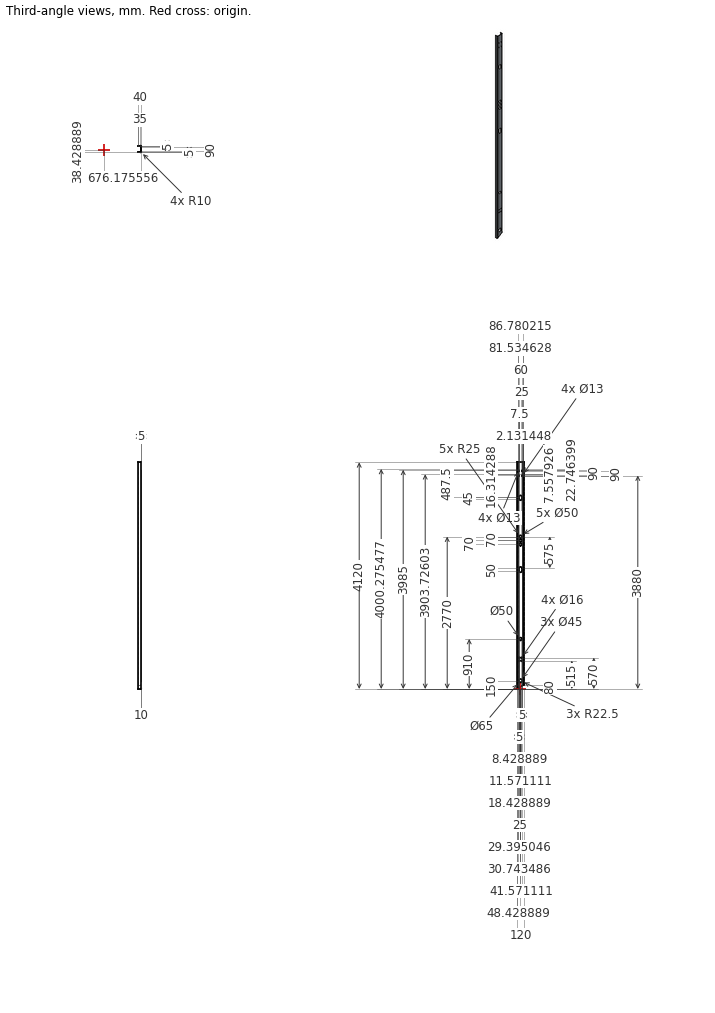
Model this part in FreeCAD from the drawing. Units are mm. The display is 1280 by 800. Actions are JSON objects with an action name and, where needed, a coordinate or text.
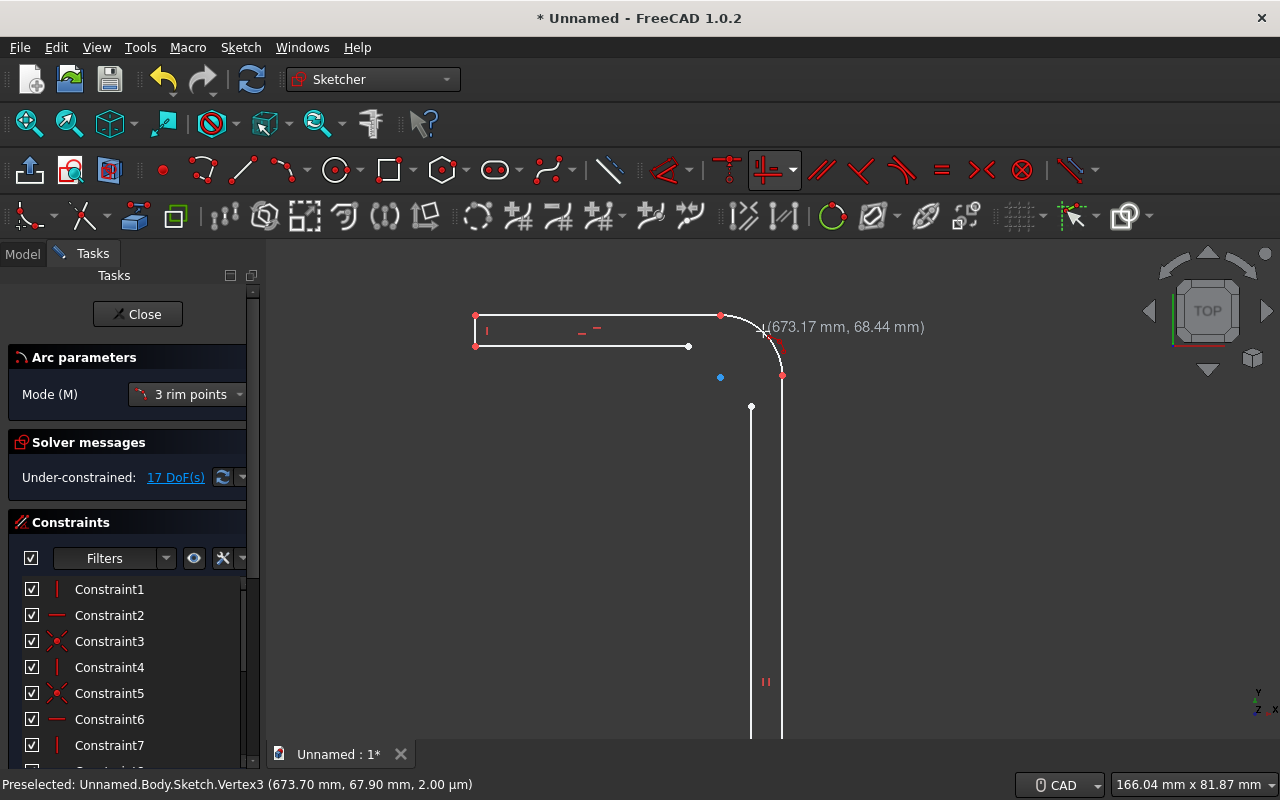
{"action": "left_click", "coordinate": [689, 346]}
{"action": "left_click", "coordinate": [751, 406]}
{"action": "left_click", "coordinate": [733, 361]}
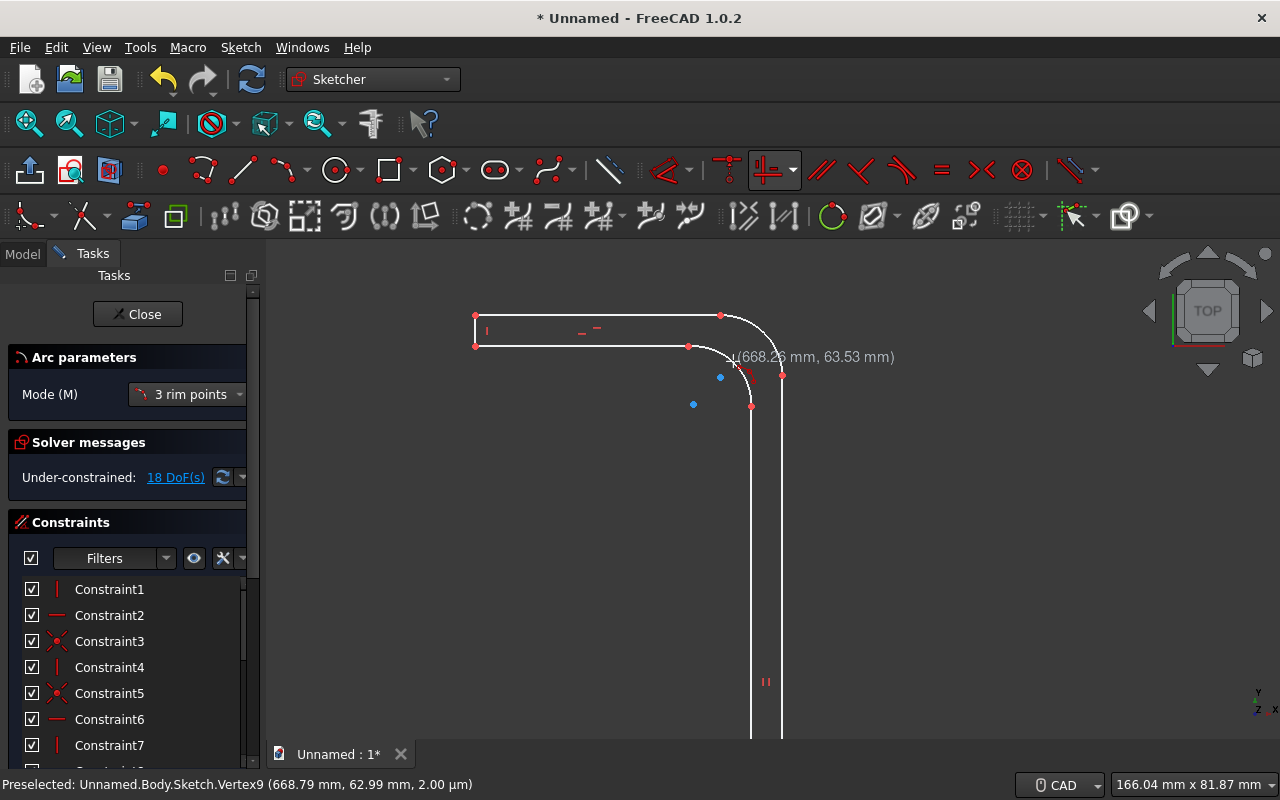
{"action": "scroll", "coordinate": [766, 334], "scroll_direction": "down", "scroll_amount": 4}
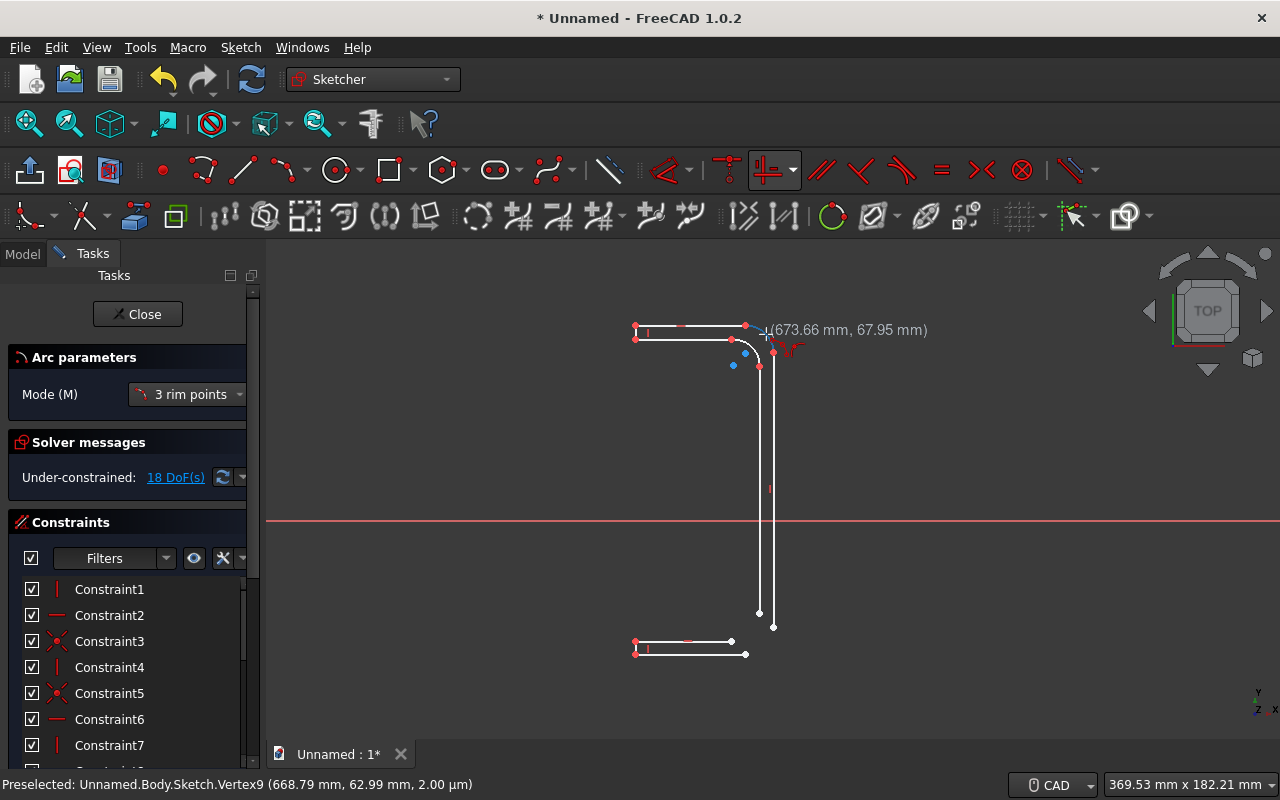
{"action": "left_click", "coordinate": [760, 614]}
{"action": "left_click", "coordinate": [732, 642]}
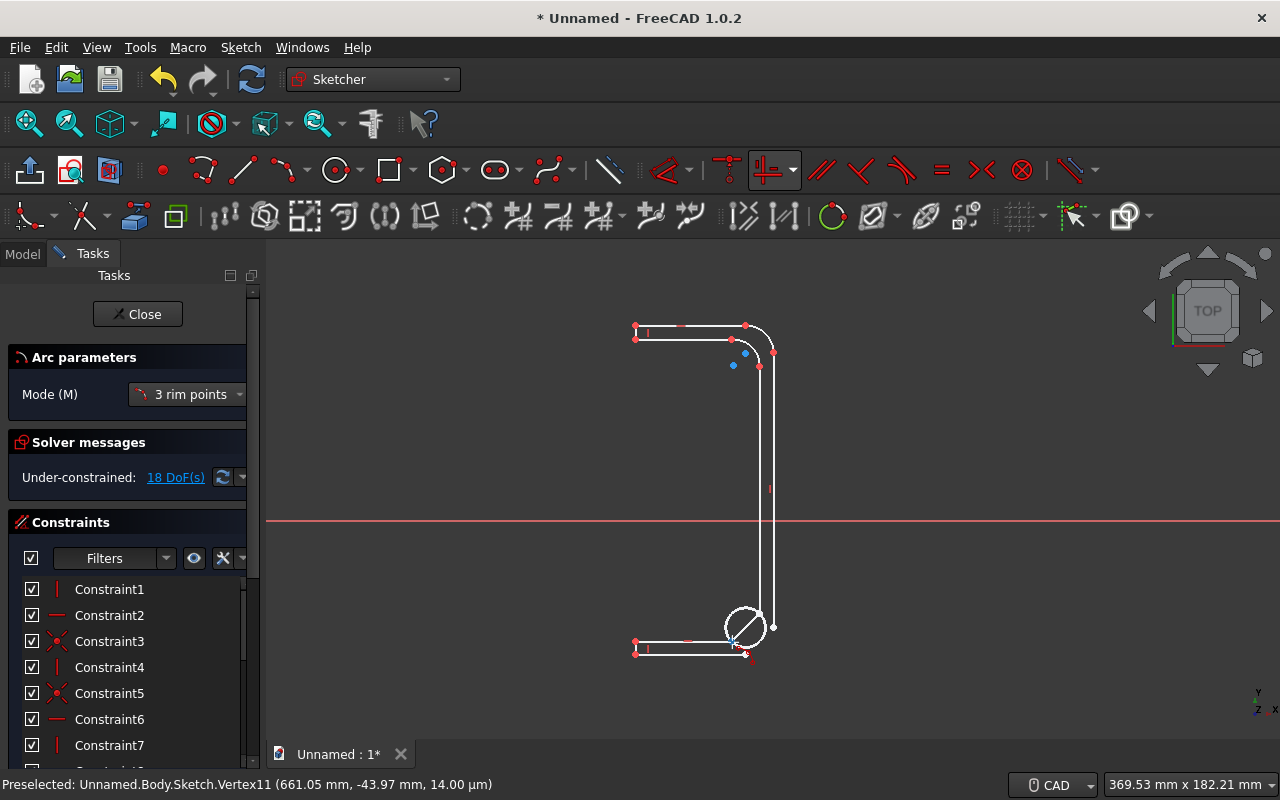
{"action": "scroll", "coordinate": [751, 632], "scroll_direction": "up", "scroll_amount": 4}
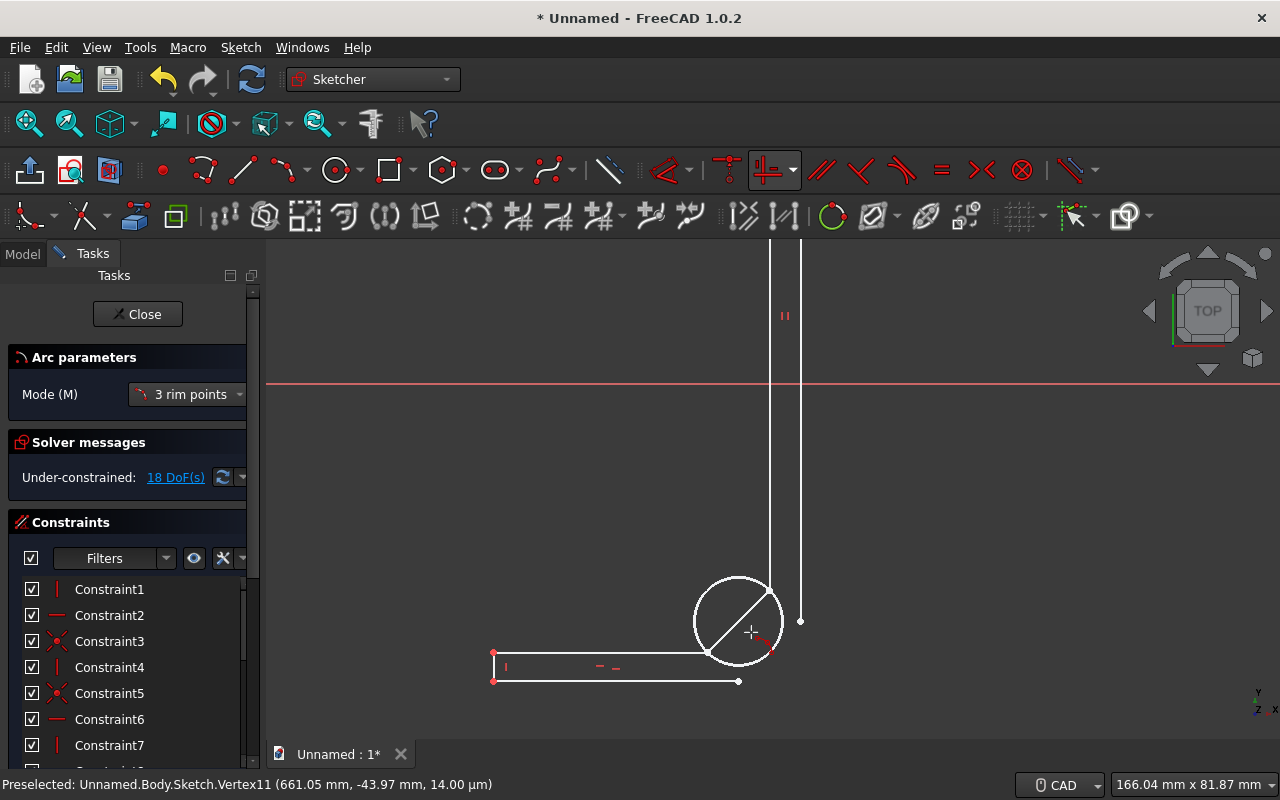
{"action": "left_click", "coordinate": [751, 631]}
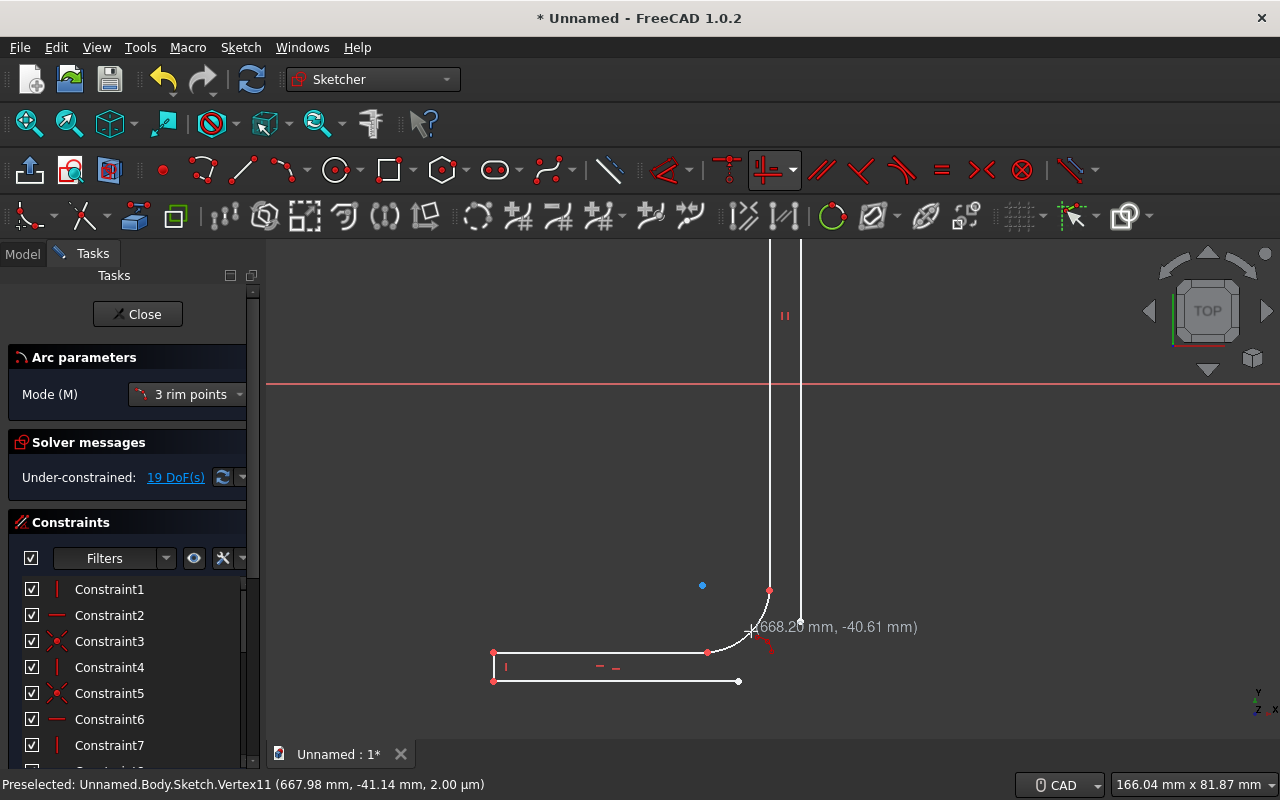
{"action": "left_click", "coordinate": [739, 681]}
{"action": "left_click", "coordinate": [801, 621]}
{"action": "left_click", "coordinate": [782, 662]}
{"action": "key", "text": "Escape"}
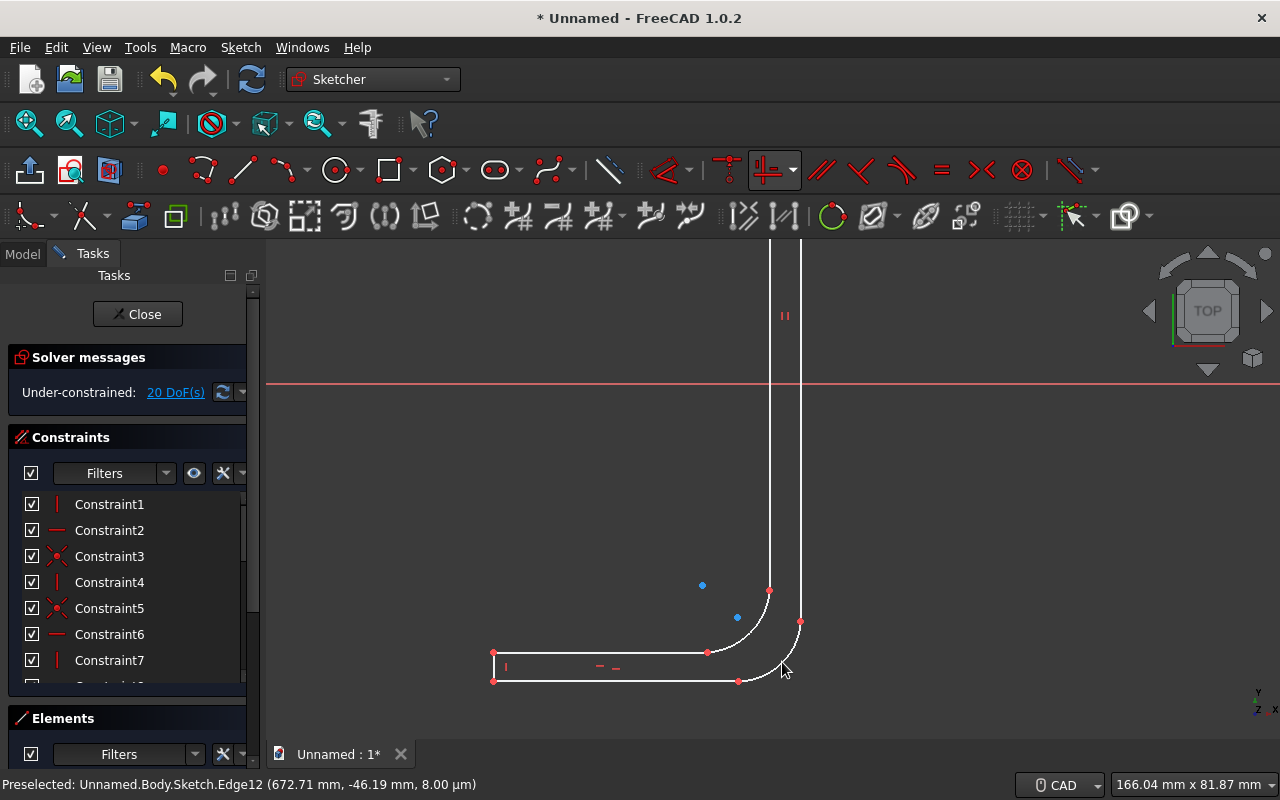
{"action": "left_click", "coordinate": [801, 438]}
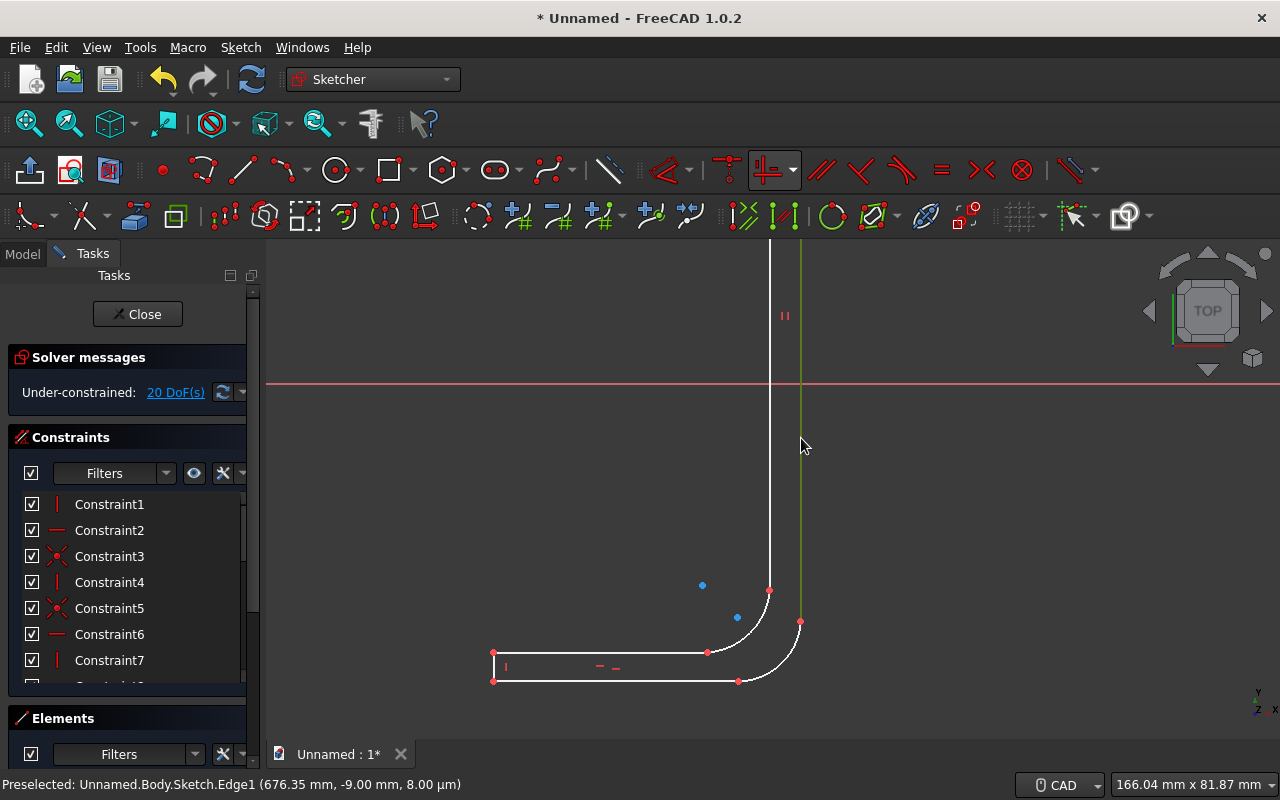
{"action": "scroll", "coordinate": [751, 632], "scroll_direction": "down", "scroll_amount": 4}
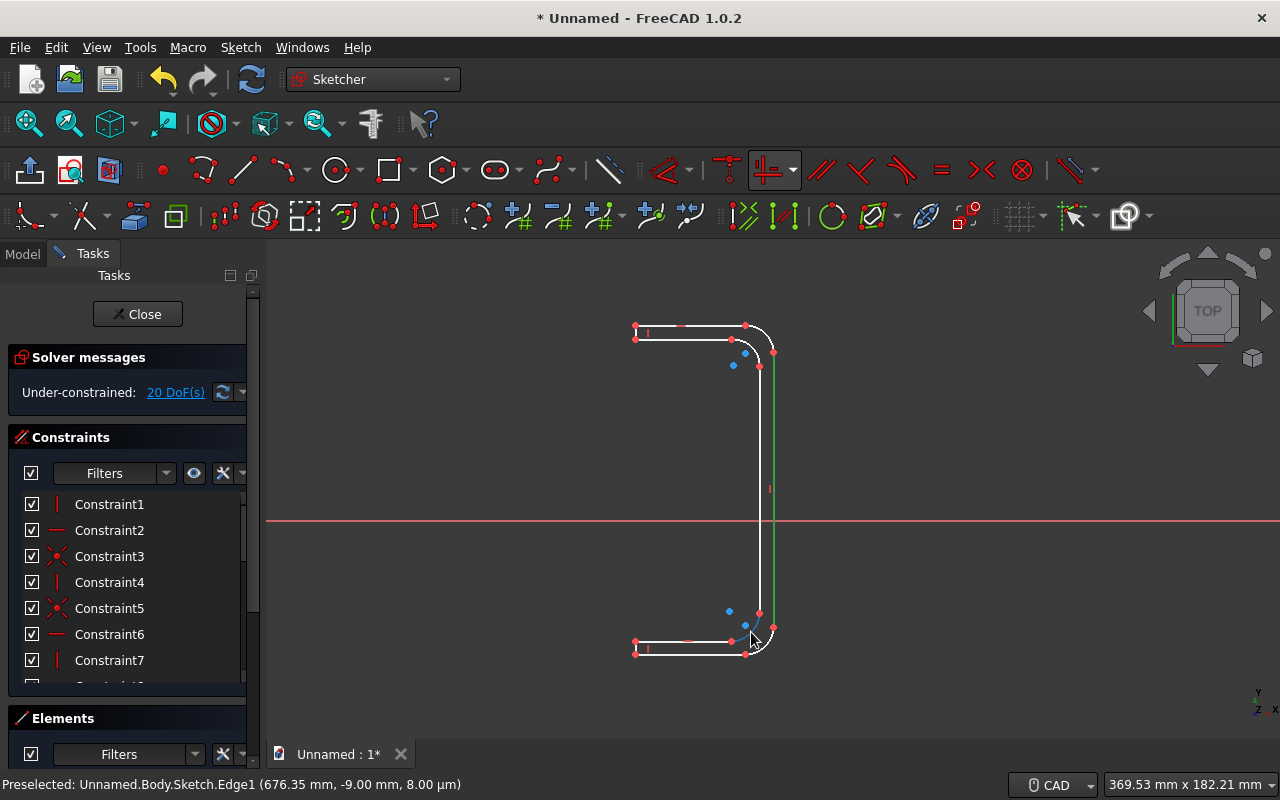
{"action": "left_click", "coordinate": [770, 340]}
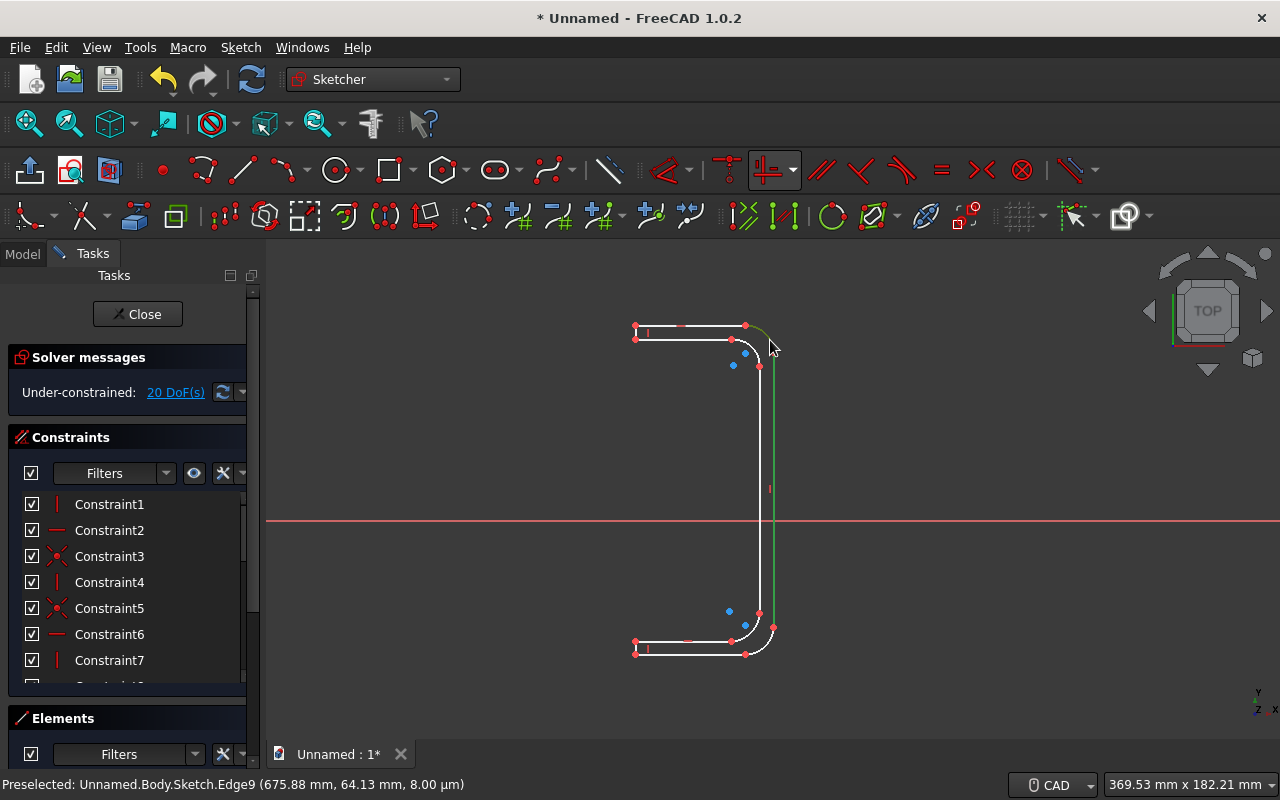
{"action": "left_click", "coordinate": [902, 170]}